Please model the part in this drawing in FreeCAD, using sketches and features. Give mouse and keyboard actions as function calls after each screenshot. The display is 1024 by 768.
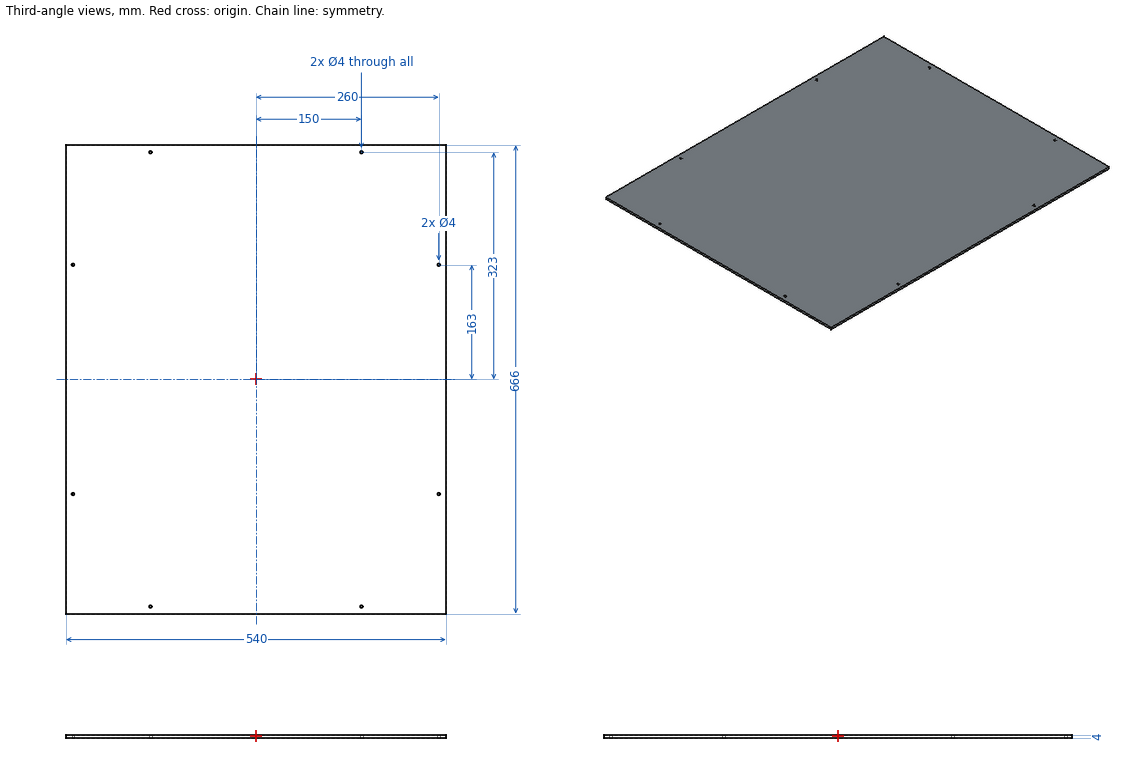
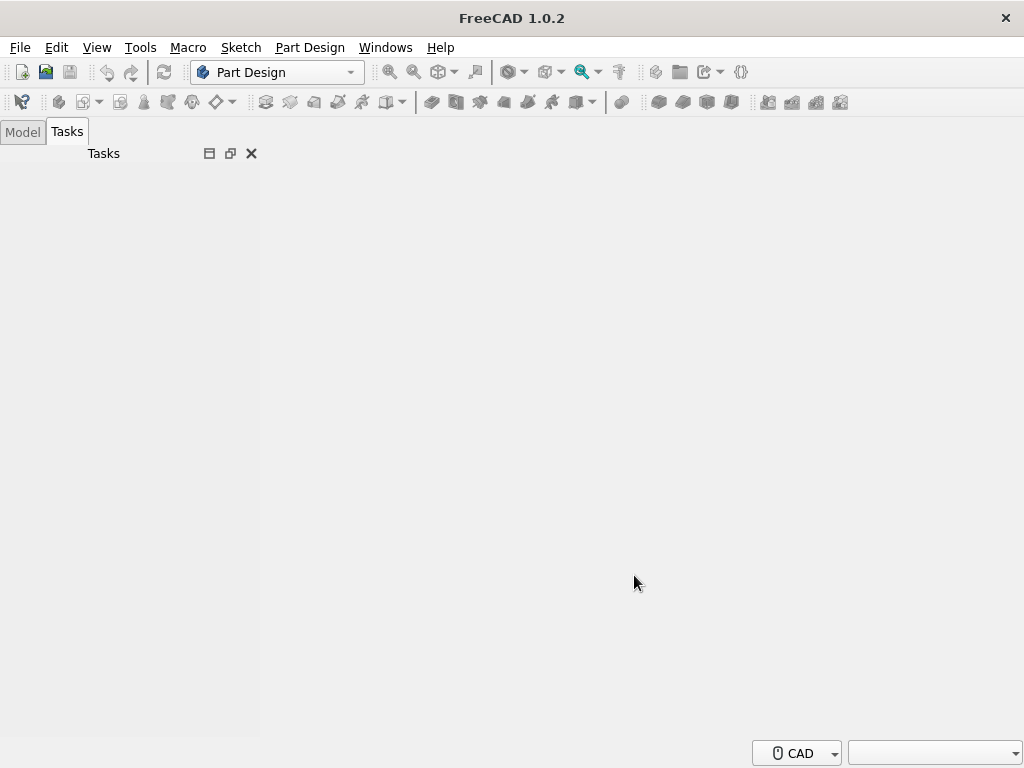
click(22, 72)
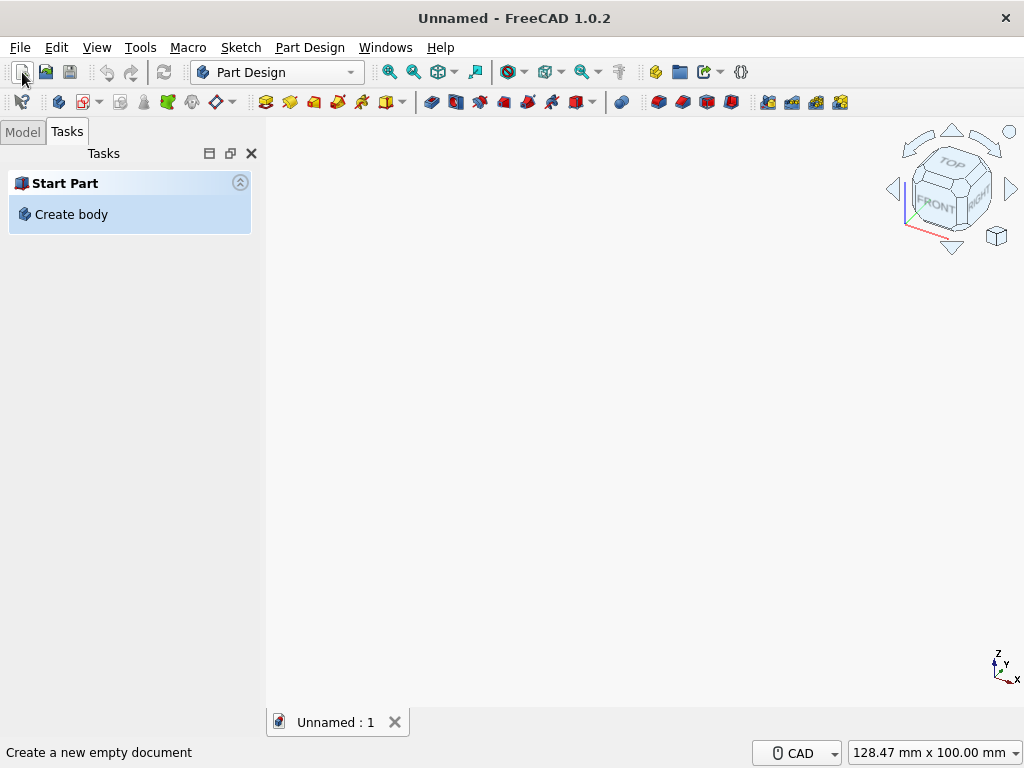
click(84, 102)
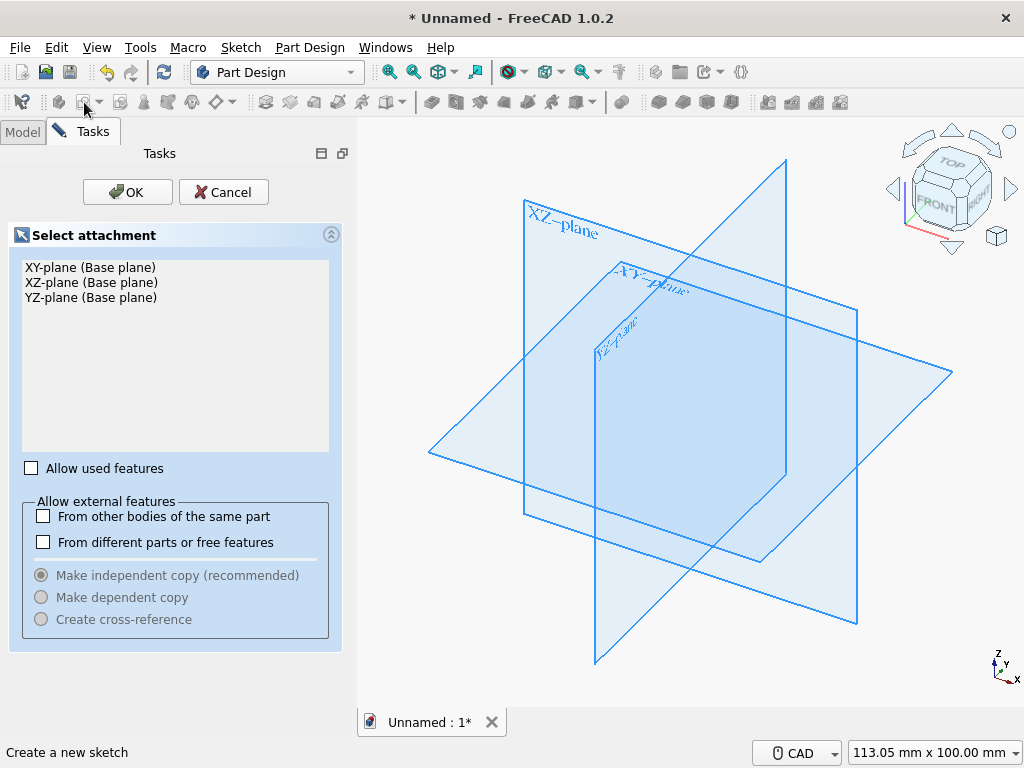
click(82, 268)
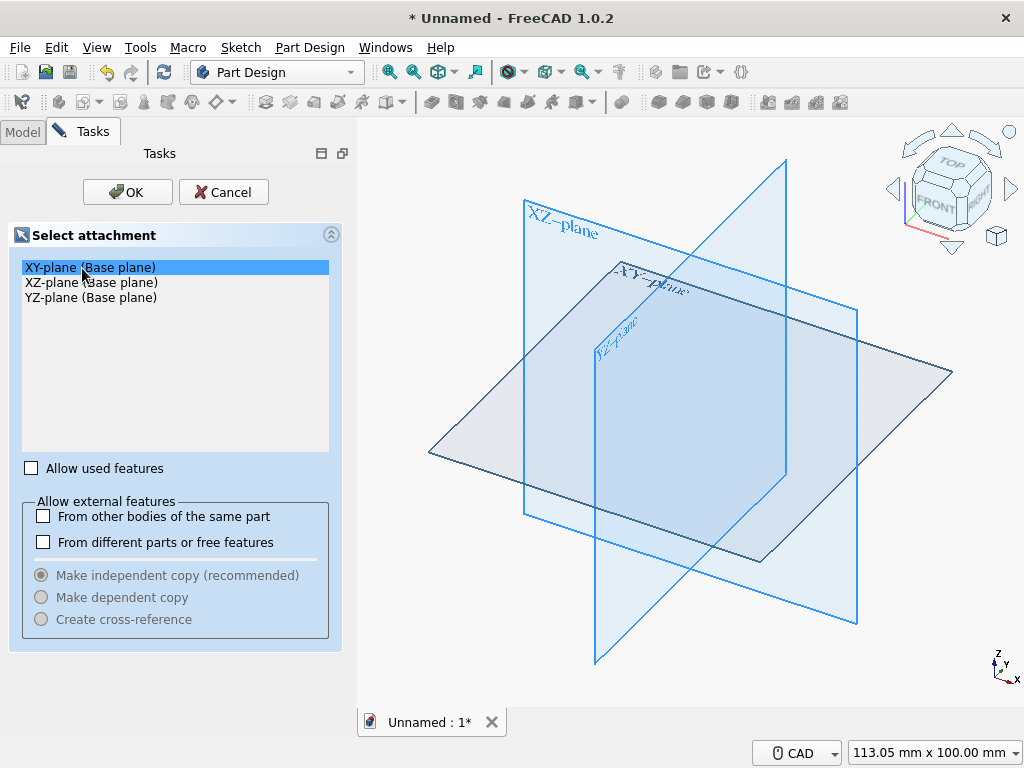
click(128, 192)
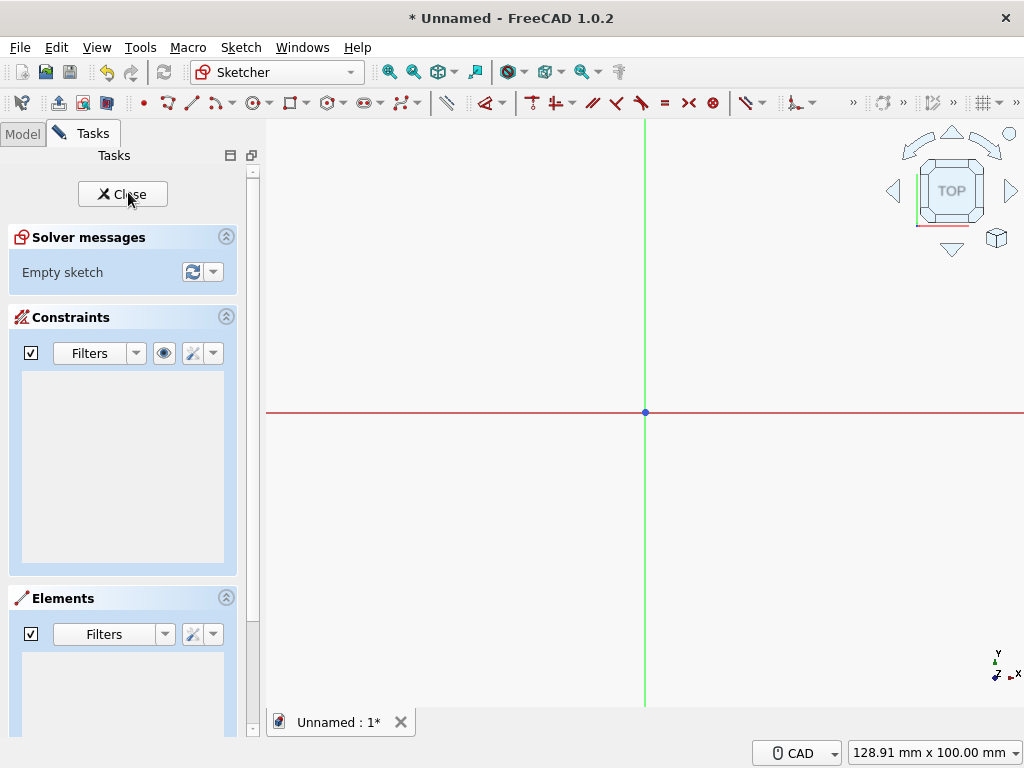
scroll(570, 413, down, 12)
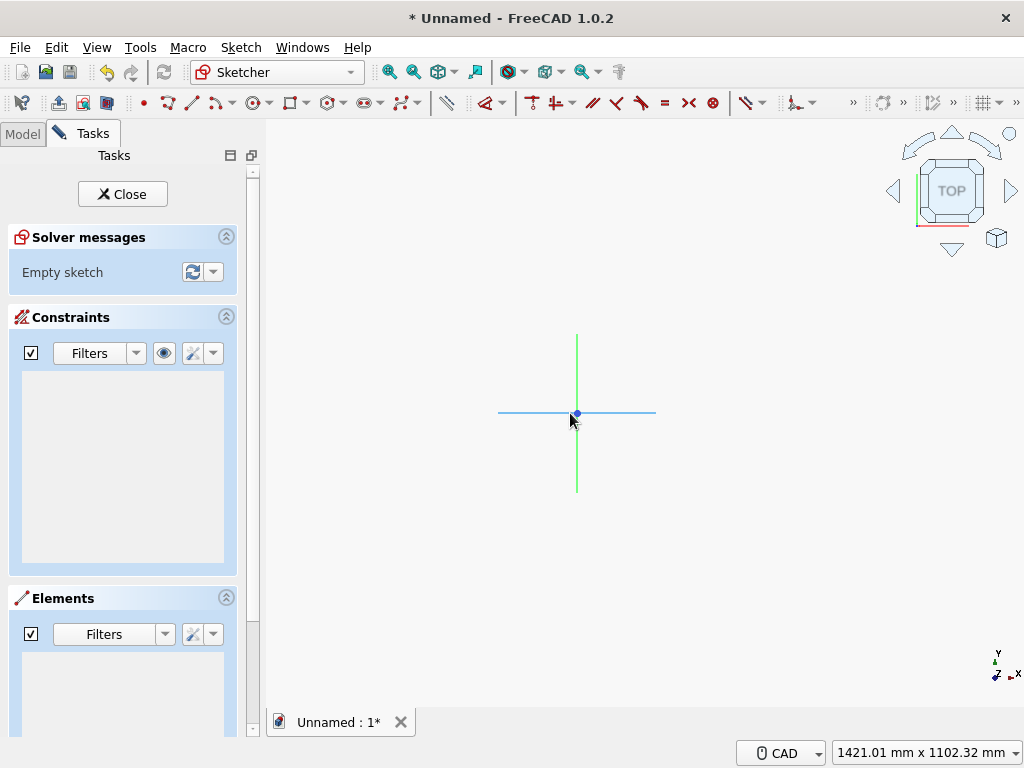
key(g)
key(v)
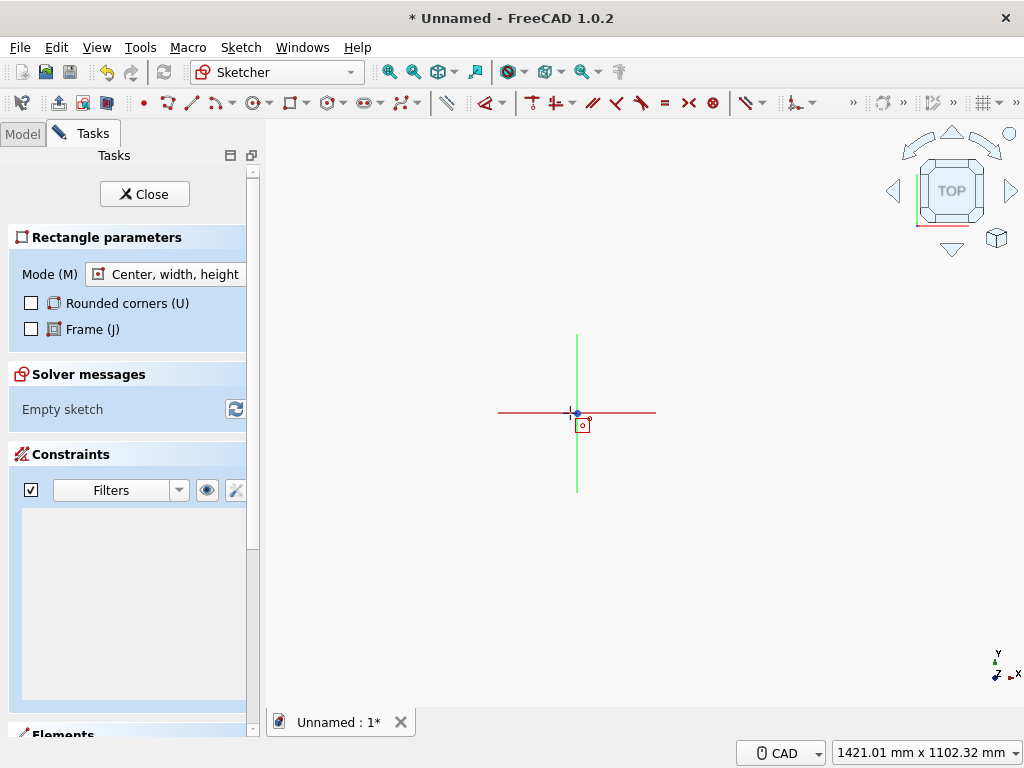
click(577, 413)
click(721, 236)
key(Escape)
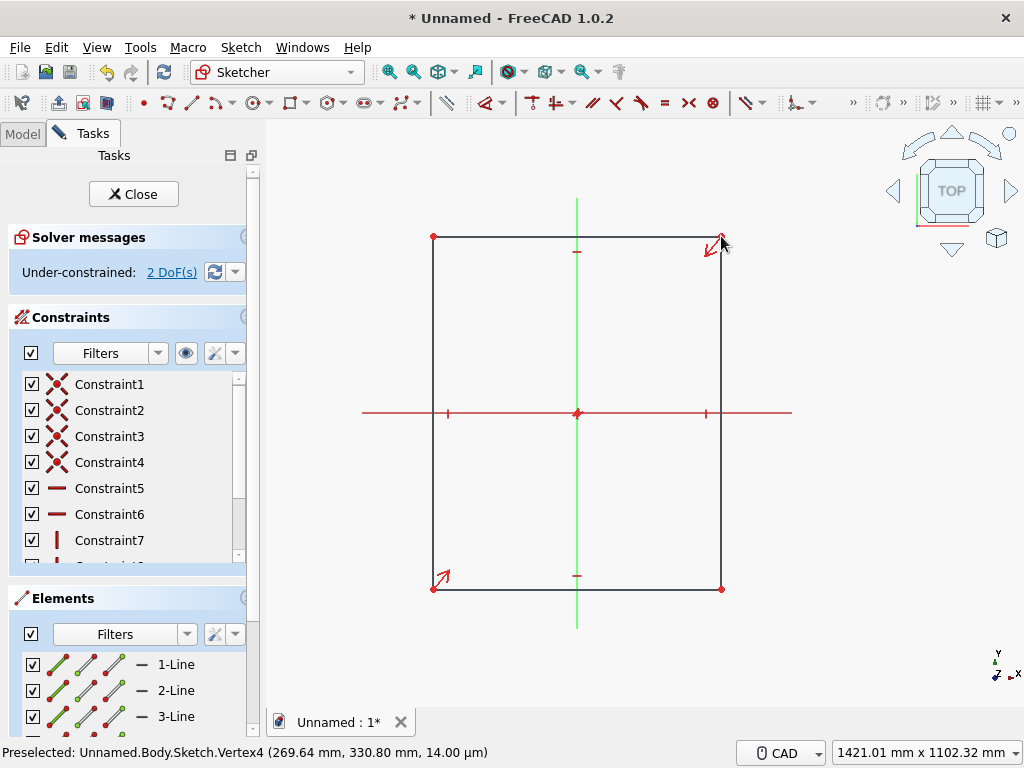
click(520, 590)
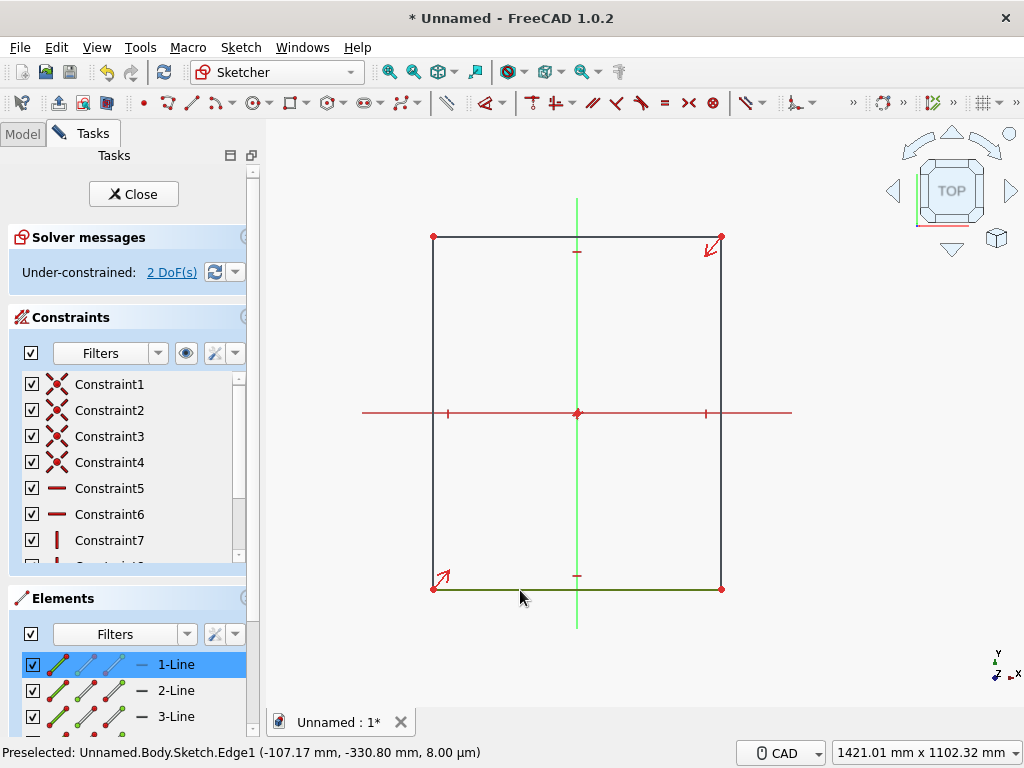
key(l)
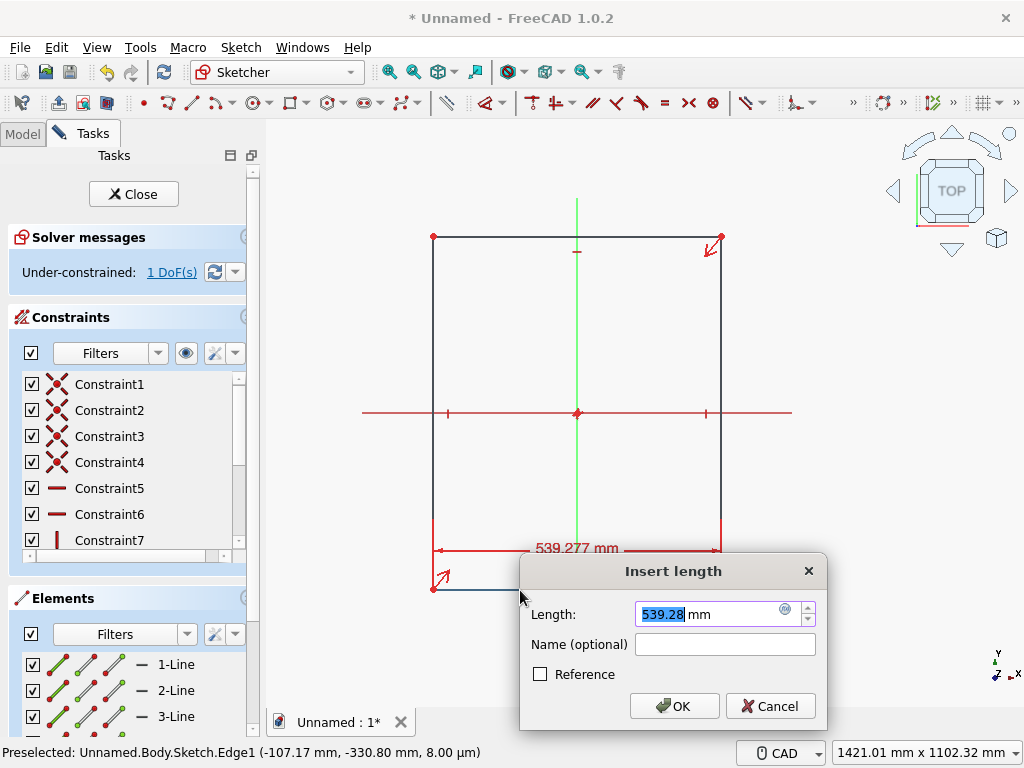
text(540)
key(Return)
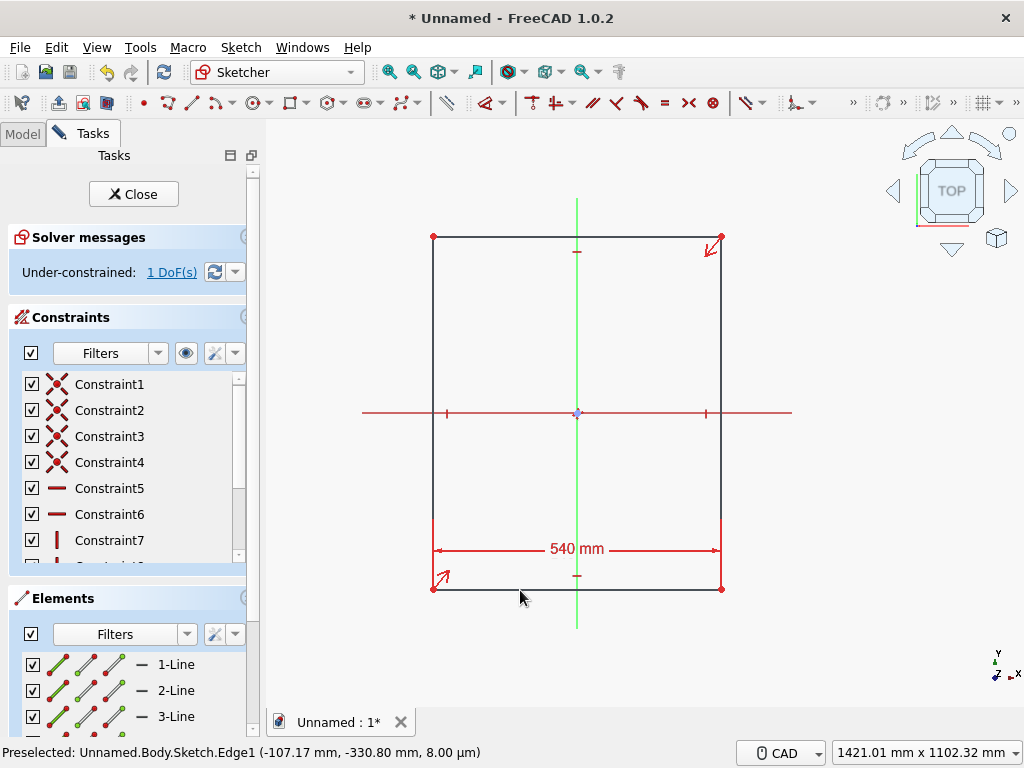
click(721, 484)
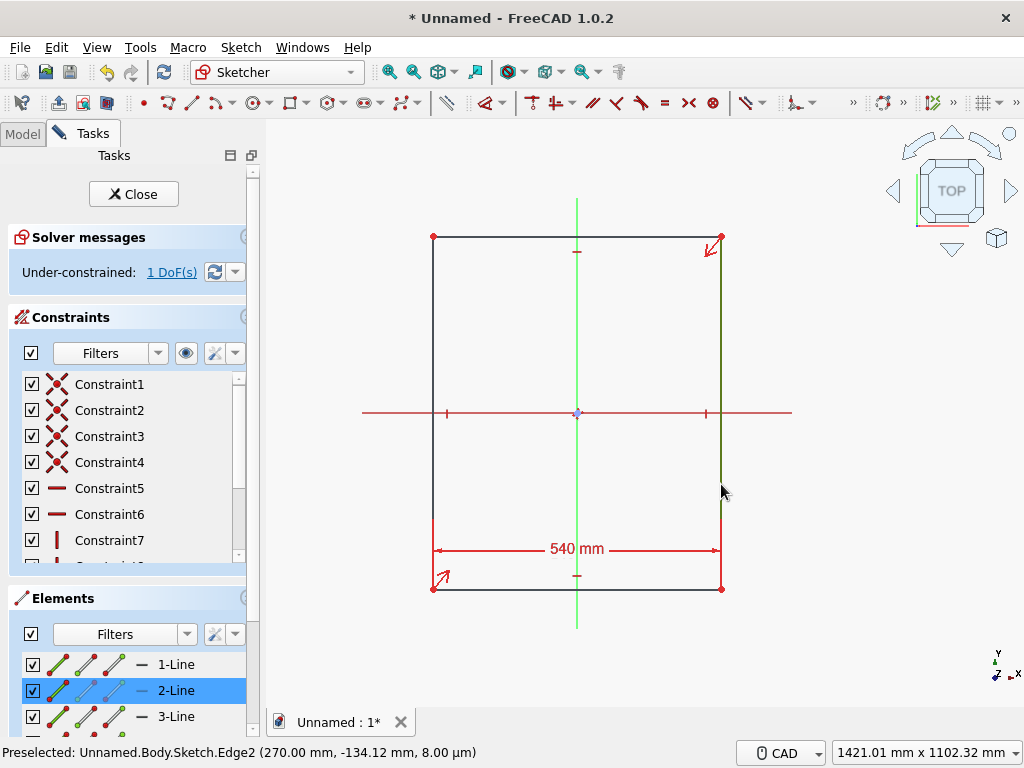
click(504, 104)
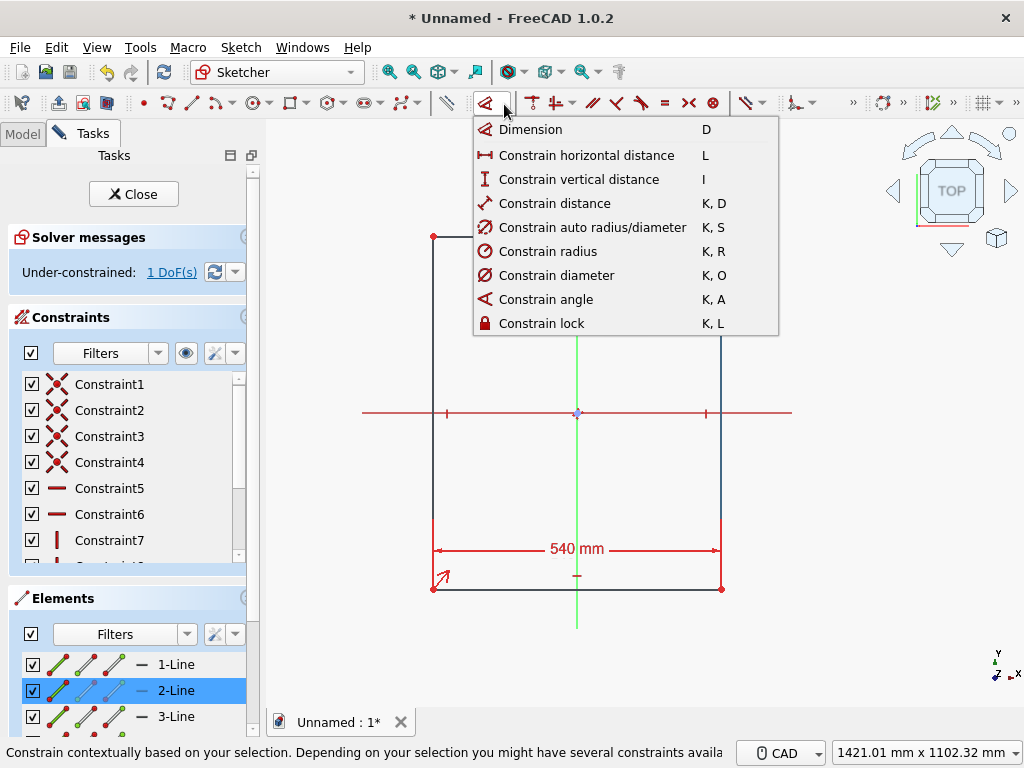
click(626, 179)